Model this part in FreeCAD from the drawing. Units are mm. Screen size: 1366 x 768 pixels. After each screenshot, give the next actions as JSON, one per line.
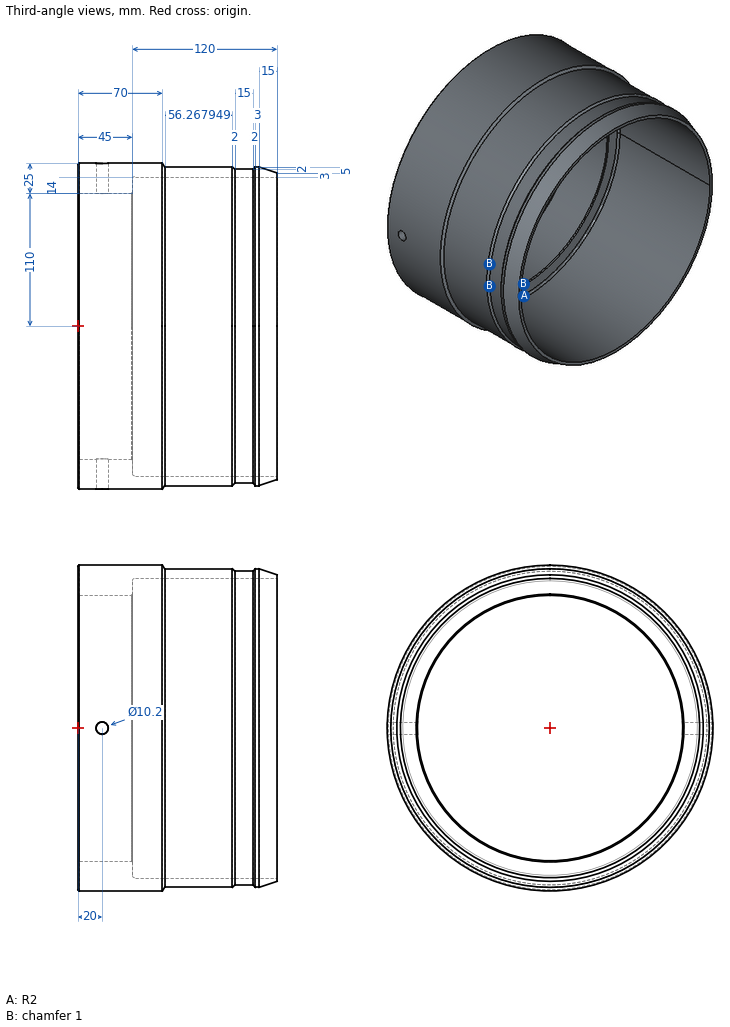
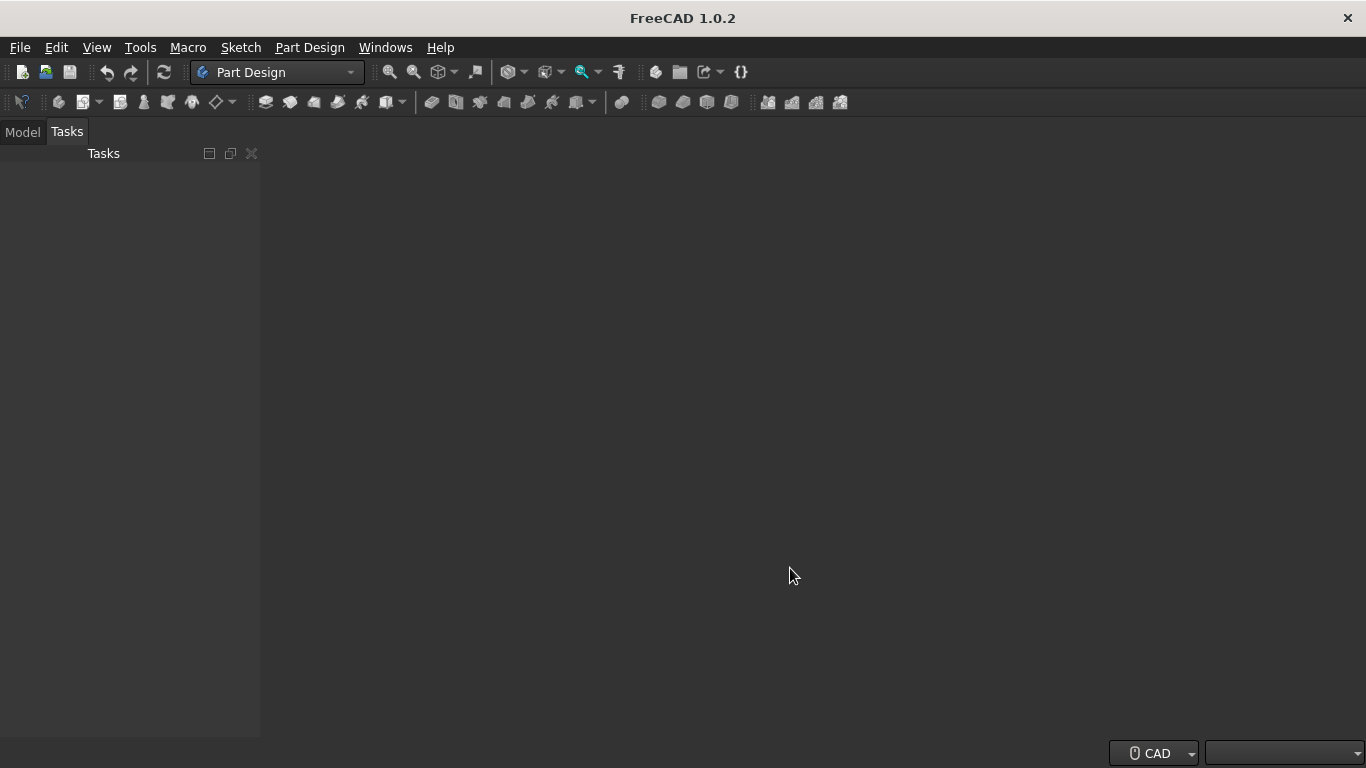
{"action": "left_click", "coordinate": [22, 72]}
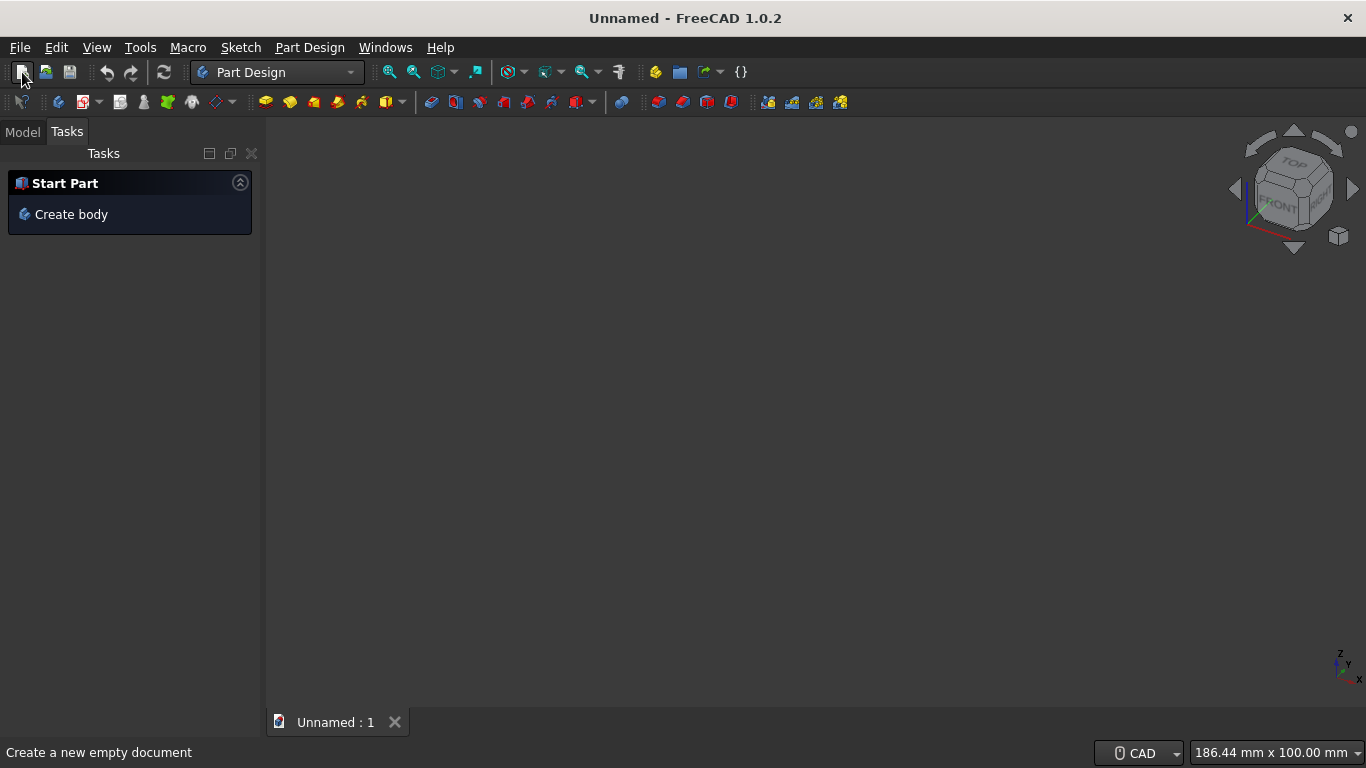
{"action": "left_click", "coordinate": [84, 102]}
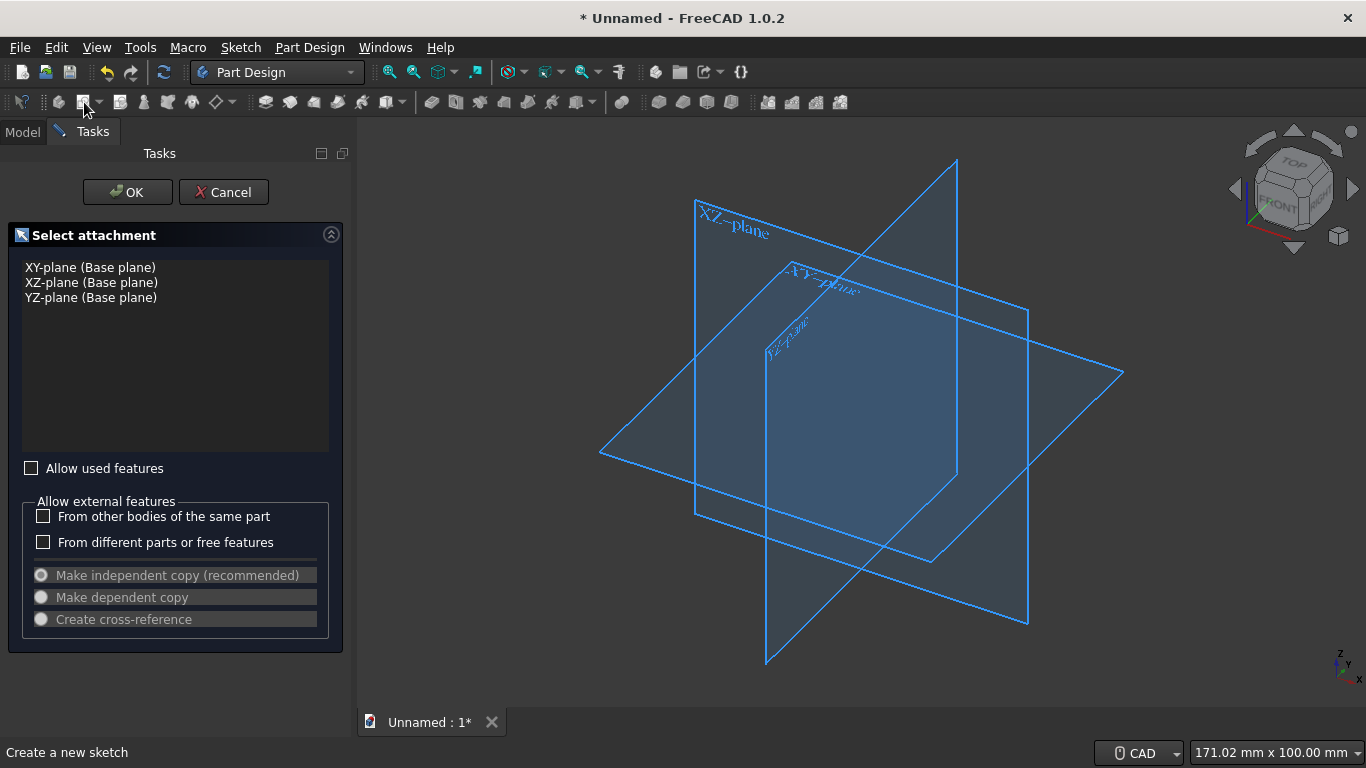
{"action": "left_click", "coordinate": [82, 268]}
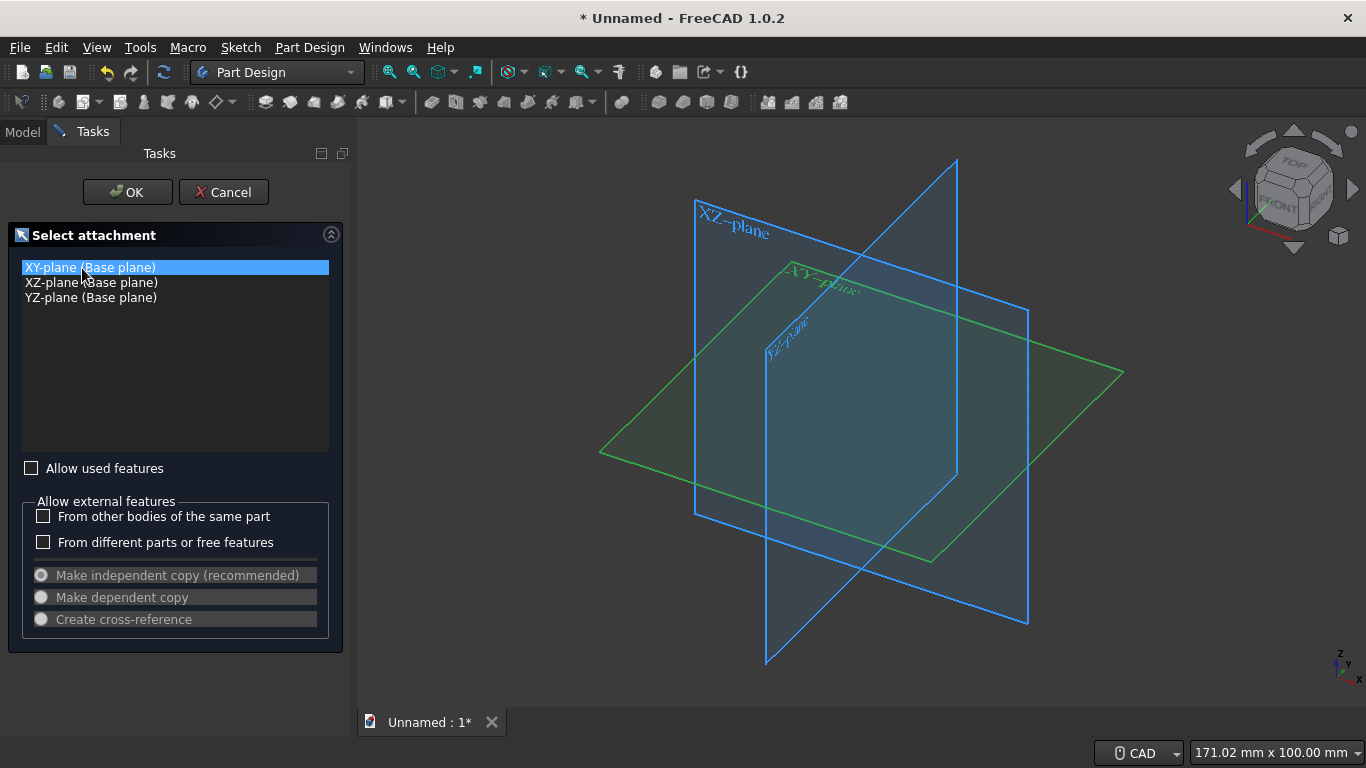
{"action": "left_click", "coordinate": [128, 192]}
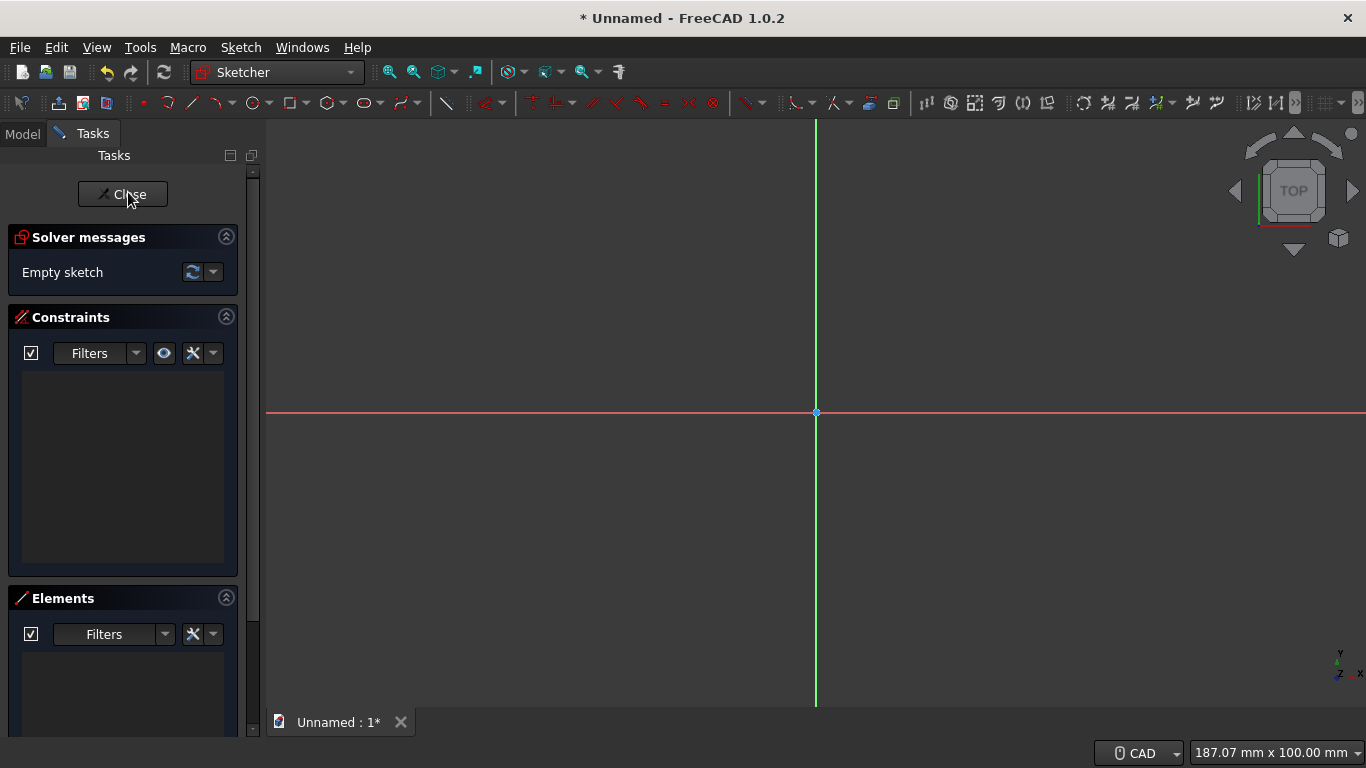
{"action": "scroll", "coordinate": [296, 679], "scroll_direction": "down", "scroll_amount": 4}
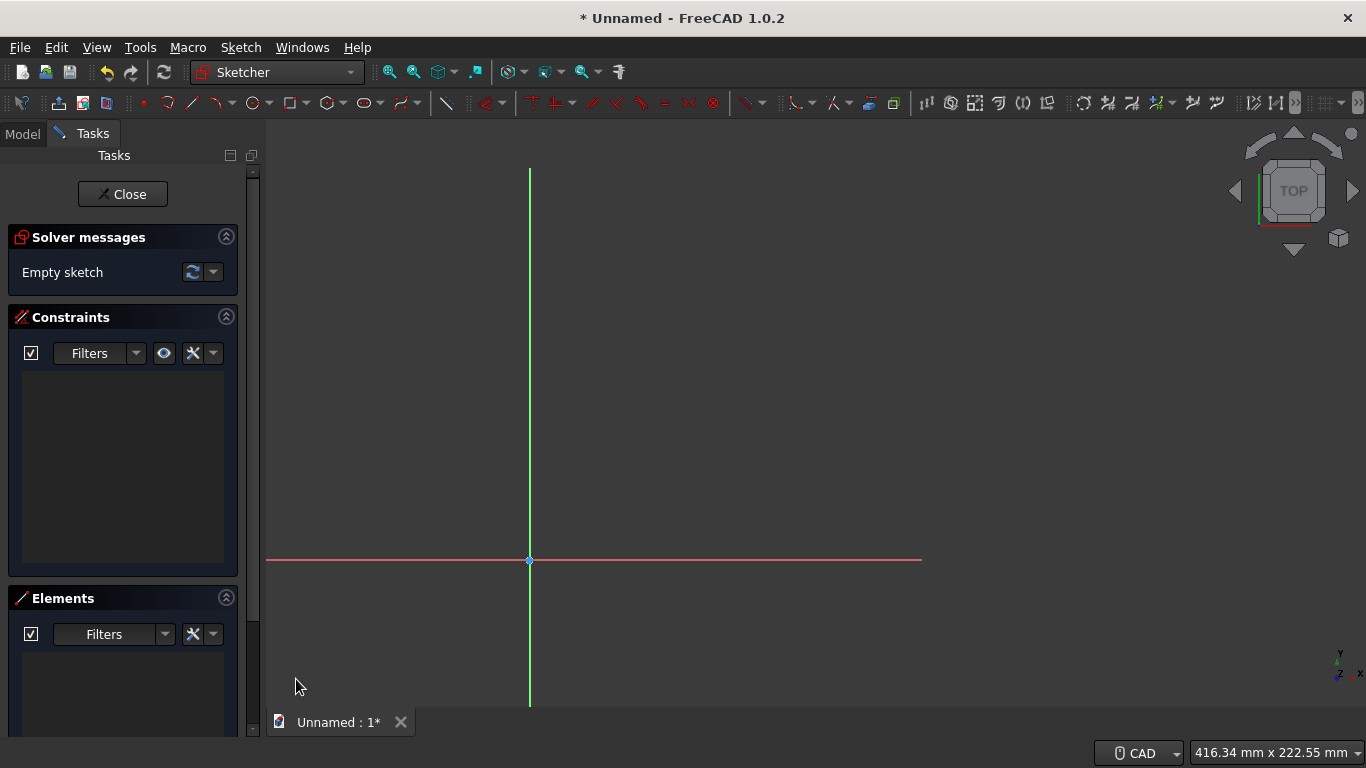
{"action": "left_click", "coordinate": [168, 104]}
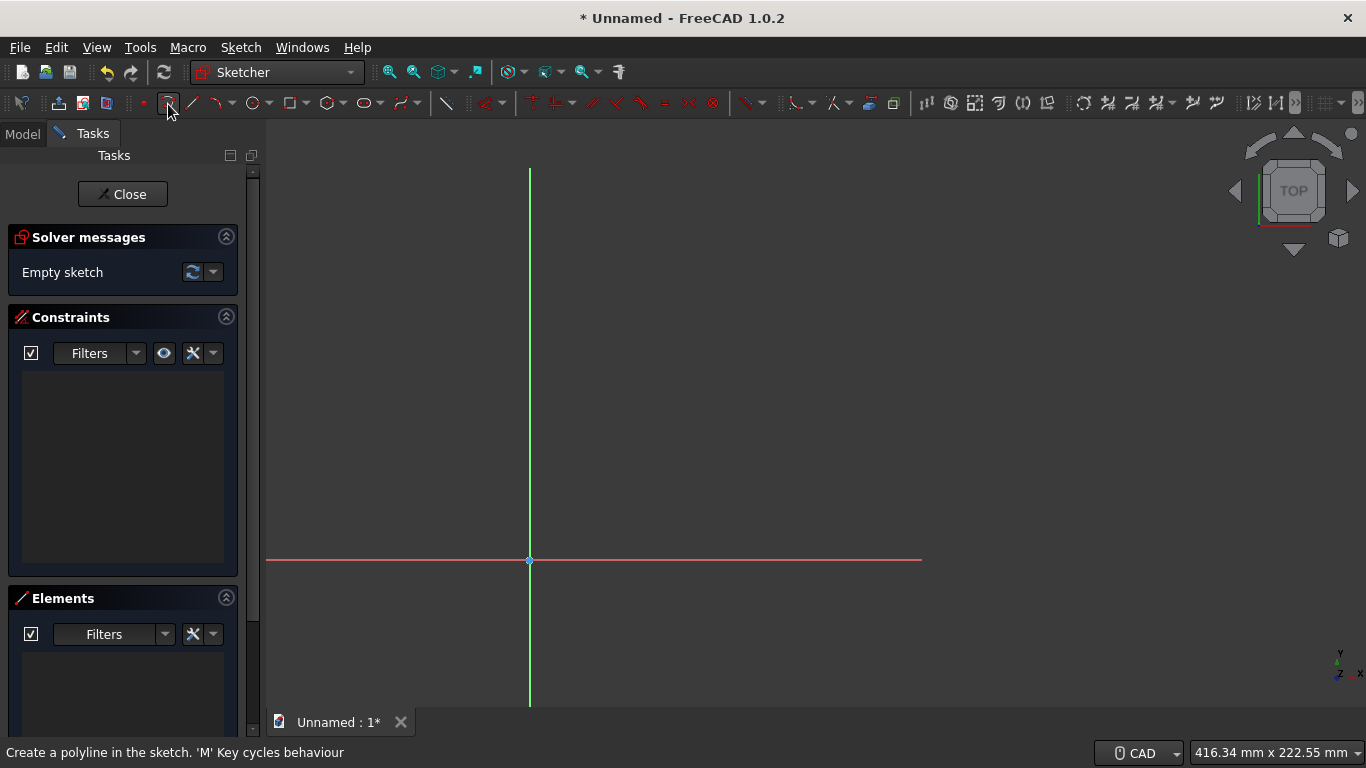
{"action": "left_click", "coordinate": [530, 269]}
{"action": "left_click", "coordinate": [649, 269]}
{"action": "left_click", "coordinate": [649, 232]}
{"action": "left_click", "coordinate": [966, 232]}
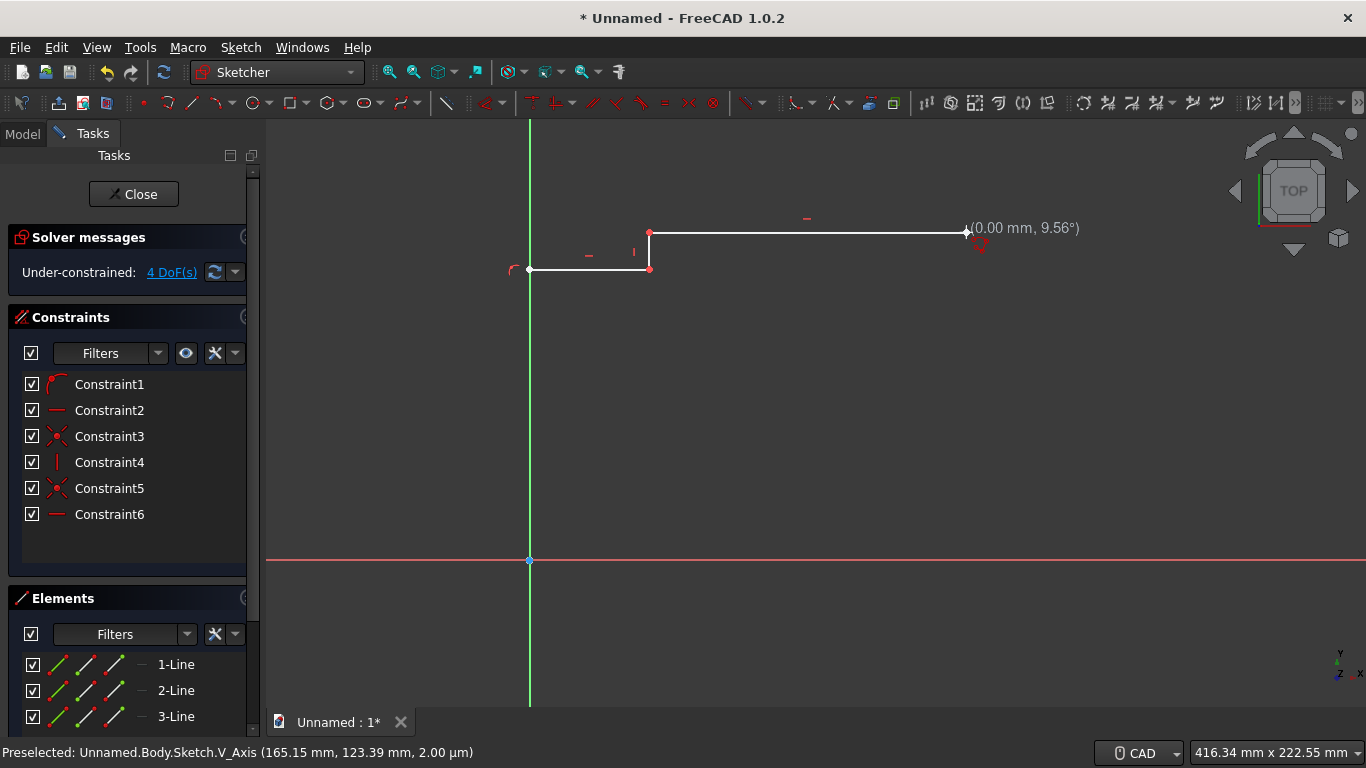
{"action": "scroll", "coordinate": [966, 224], "scroll_direction": "up", "scroll_amount": 4}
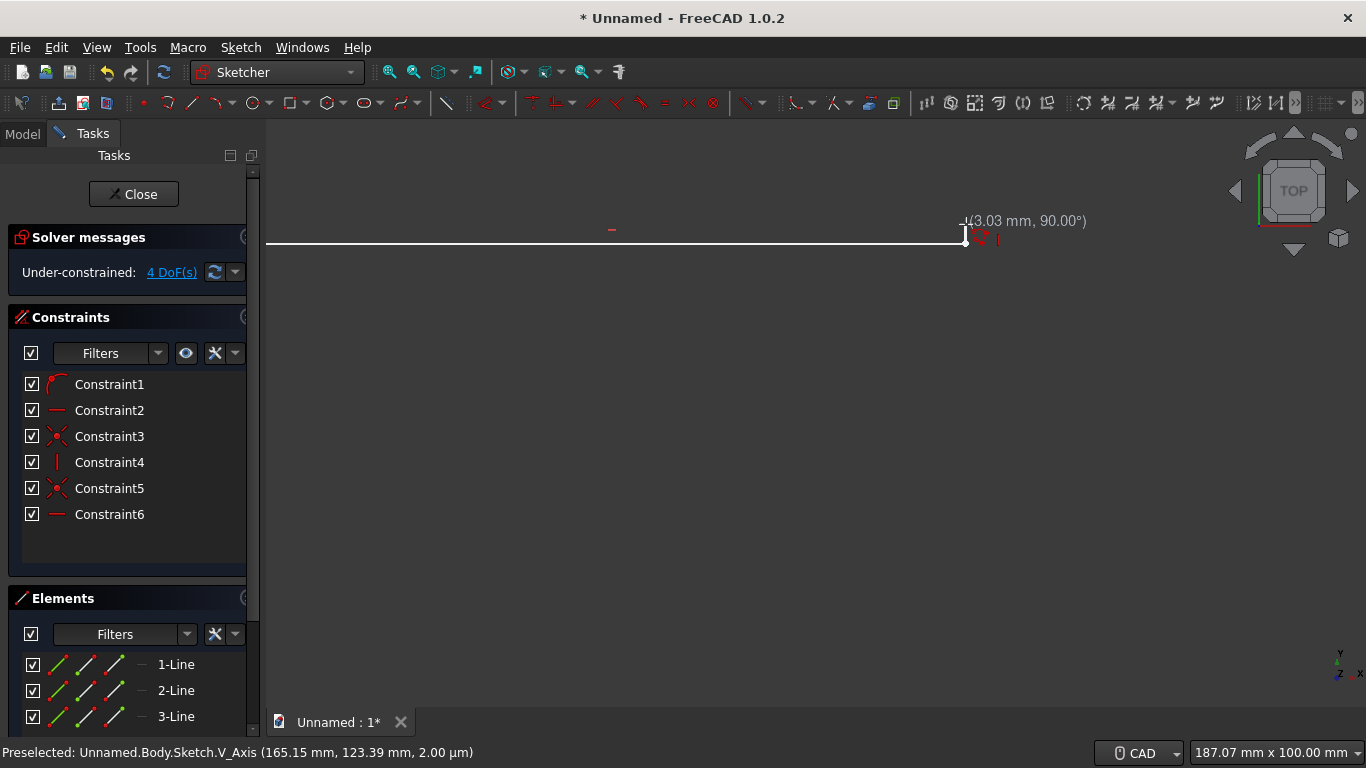
{"action": "left_click", "coordinate": [965, 225]}
{"action": "left_click", "coordinate": [876, 195]}
{"action": "left_click", "coordinate": [859, 195]}
{"action": "left_click", "coordinate": [847, 207]}
{"action": "left_click", "coordinate": [759, 207]}
{"action": "left_click", "coordinate": [747, 195]}
{"action": "left_click", "coordinate": [416, 195]}
{"action": "left_click", "coordinate": [406, 178]}